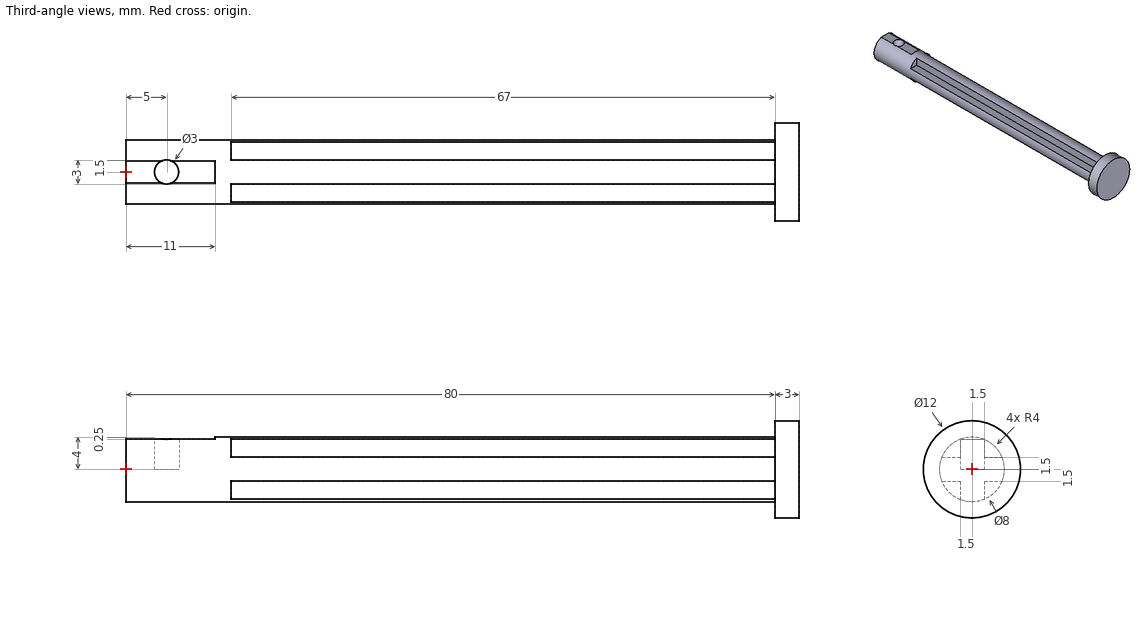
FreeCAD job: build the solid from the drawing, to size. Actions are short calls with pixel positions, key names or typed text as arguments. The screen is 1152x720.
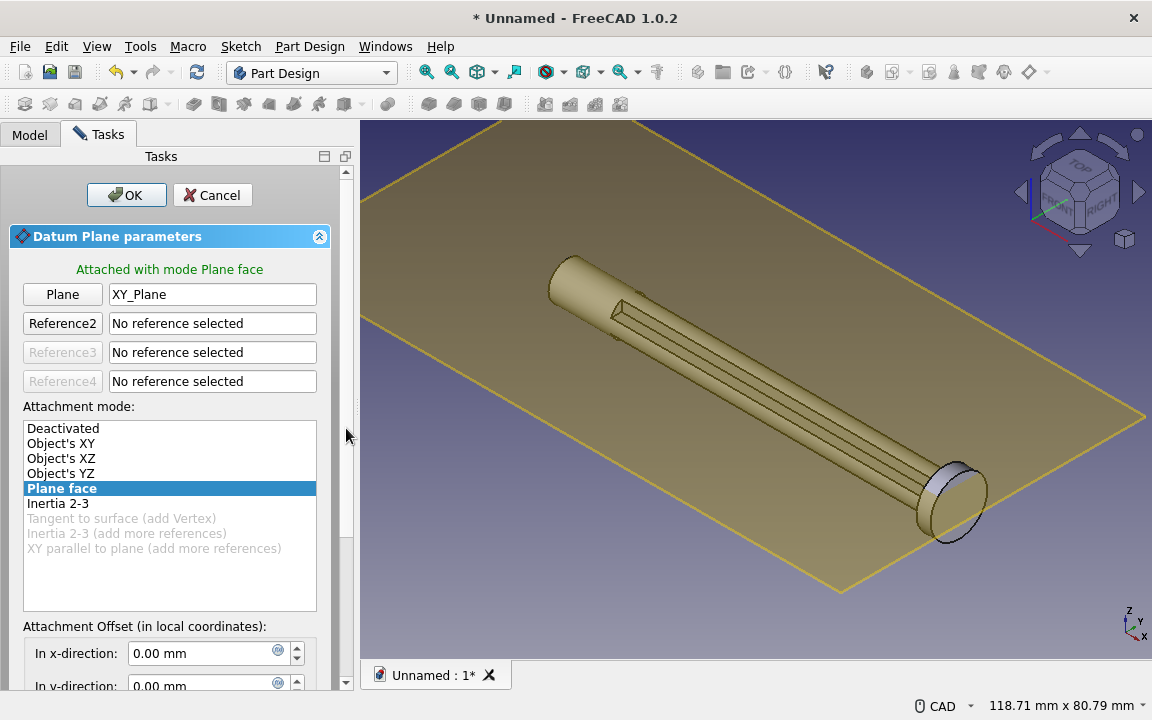
click(127, 195)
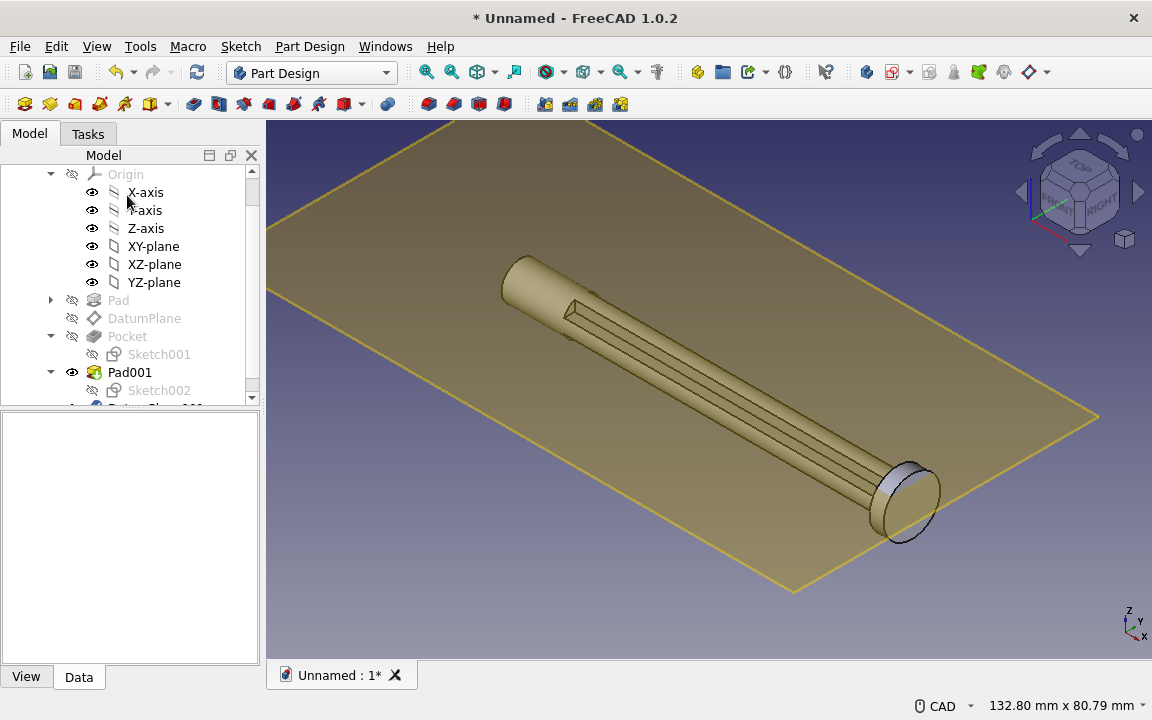
scroll(141, 278, down, 3)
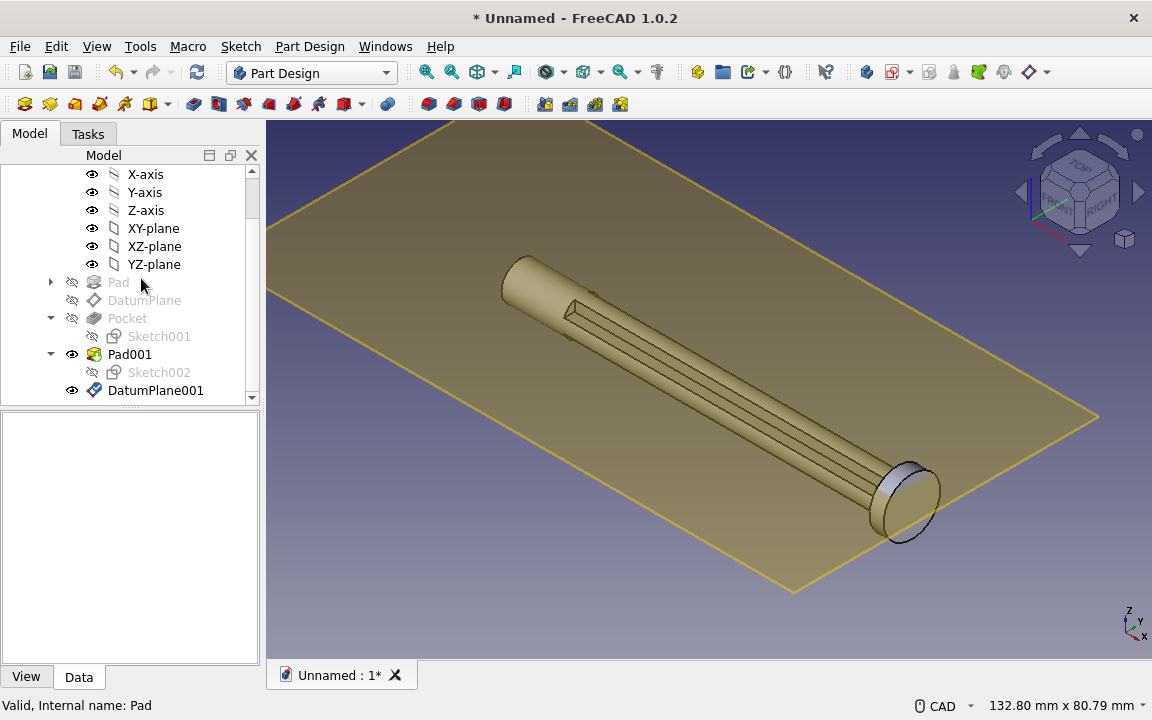
click(117, 390)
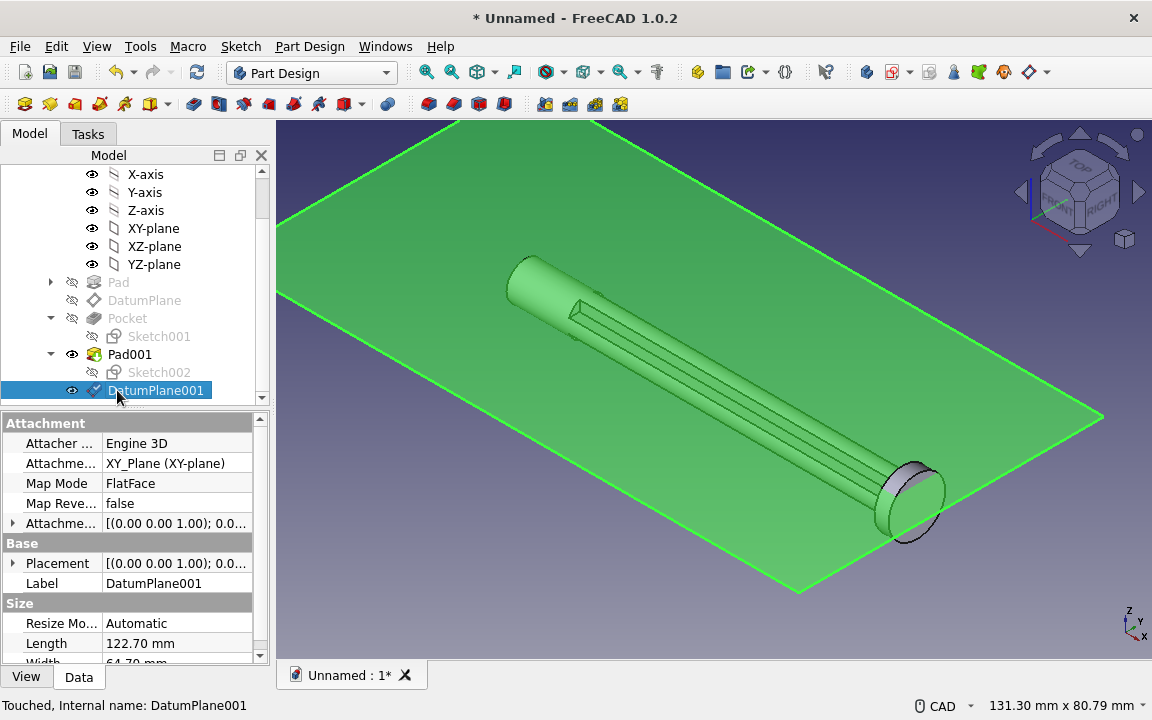
click(892, 72)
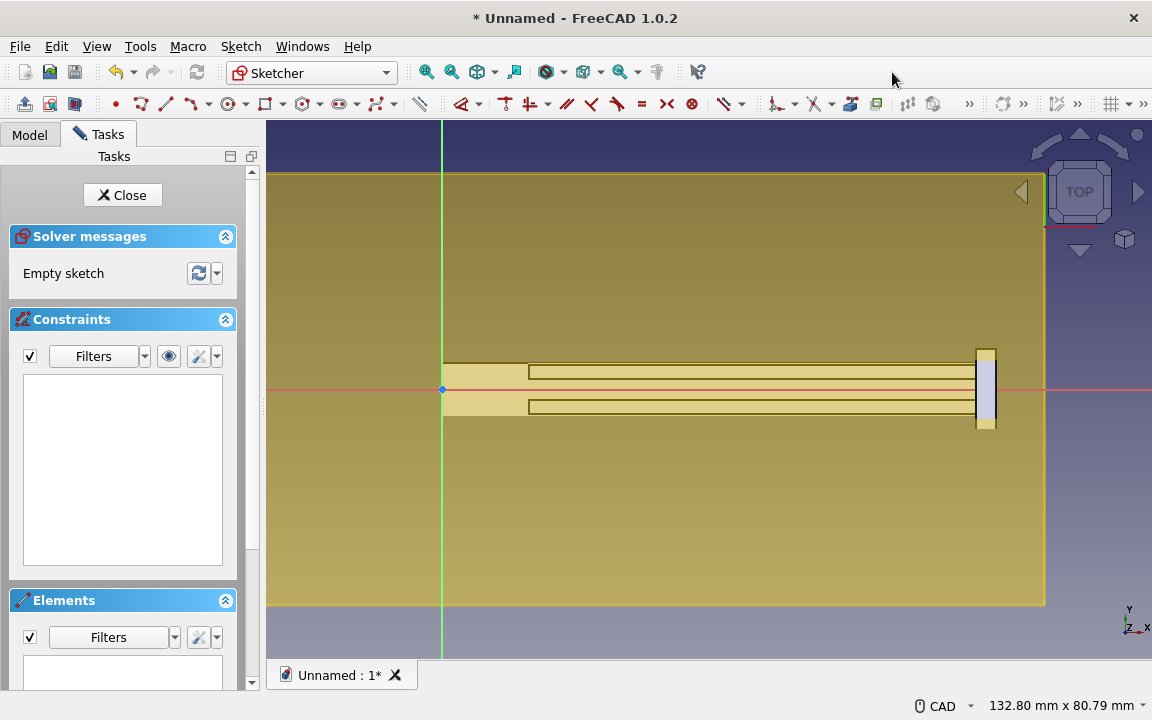
key(q)
key(s)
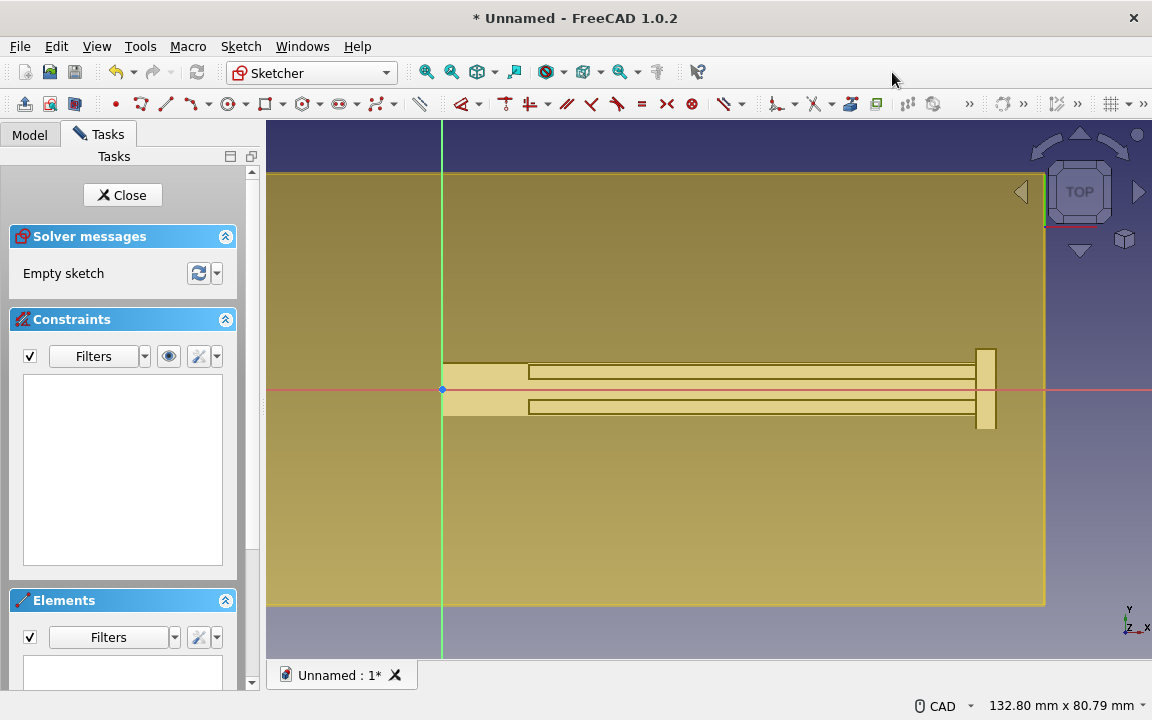
scroll(446, 390, up, 12)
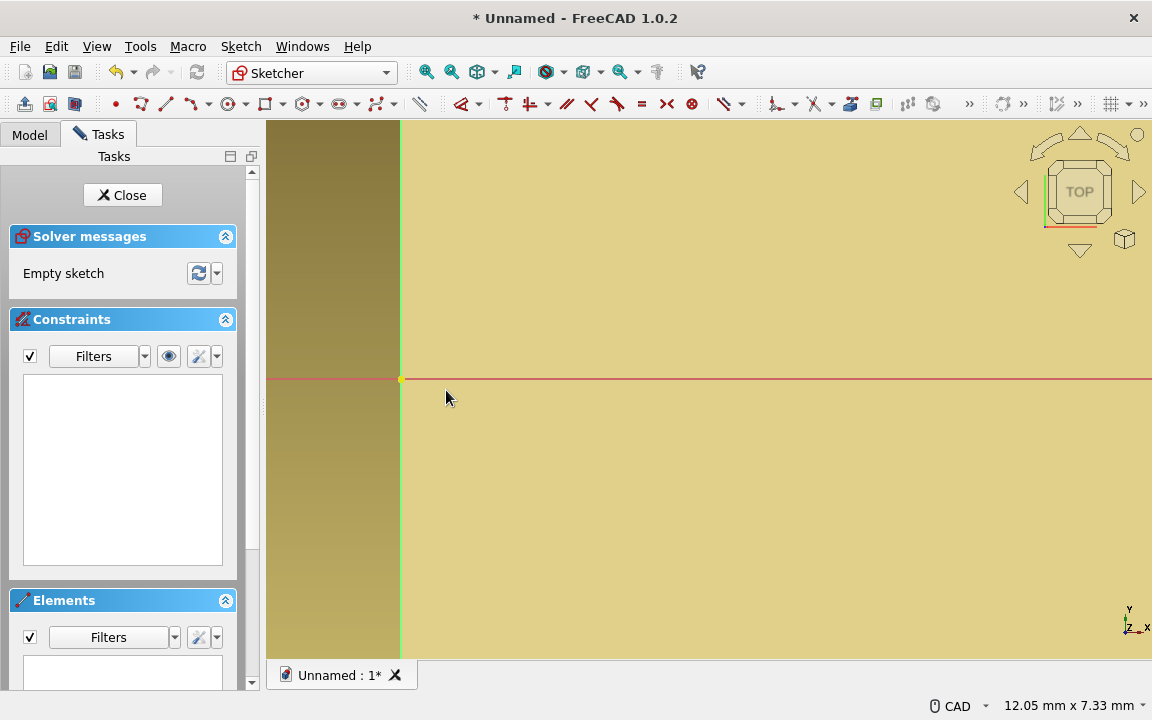
key(g)
key(c)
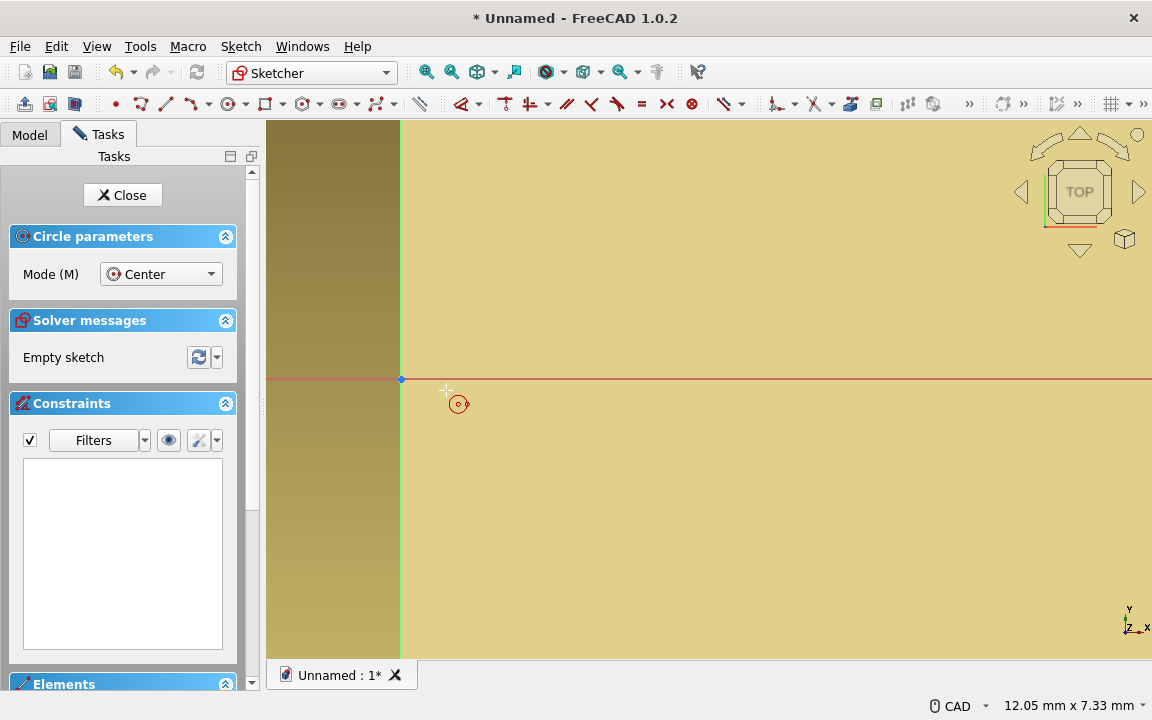
click(769, 379)
move(847, 301)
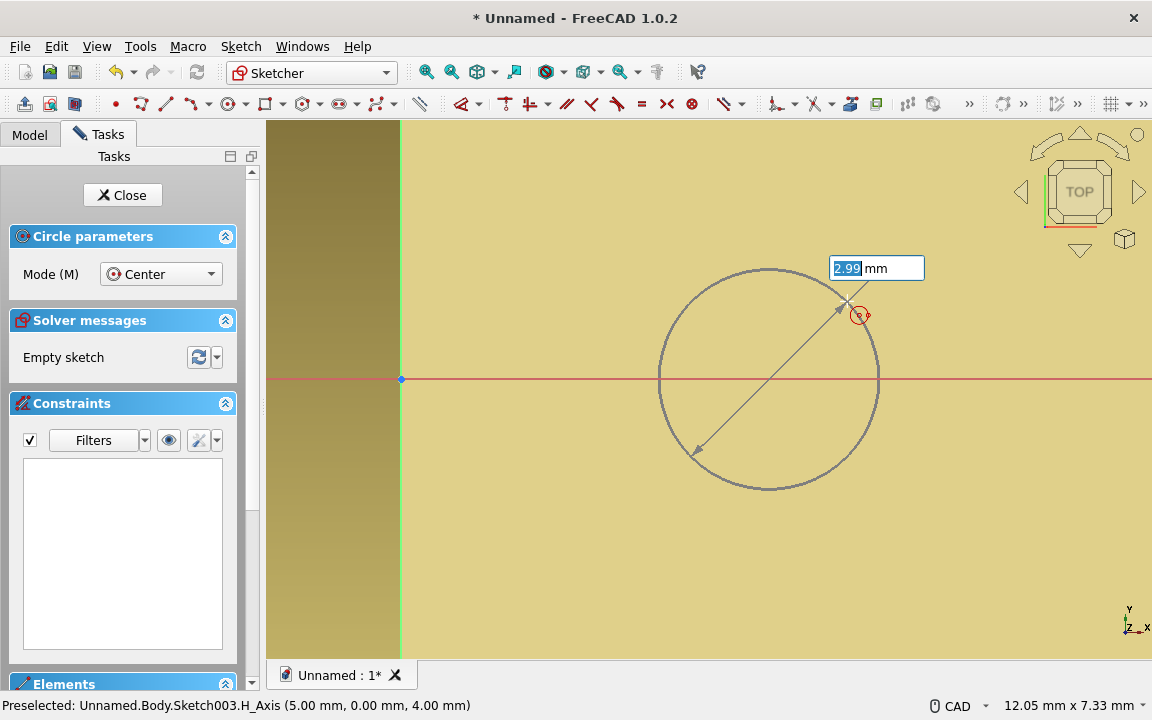
text(3)
key(Return)
key(Escape)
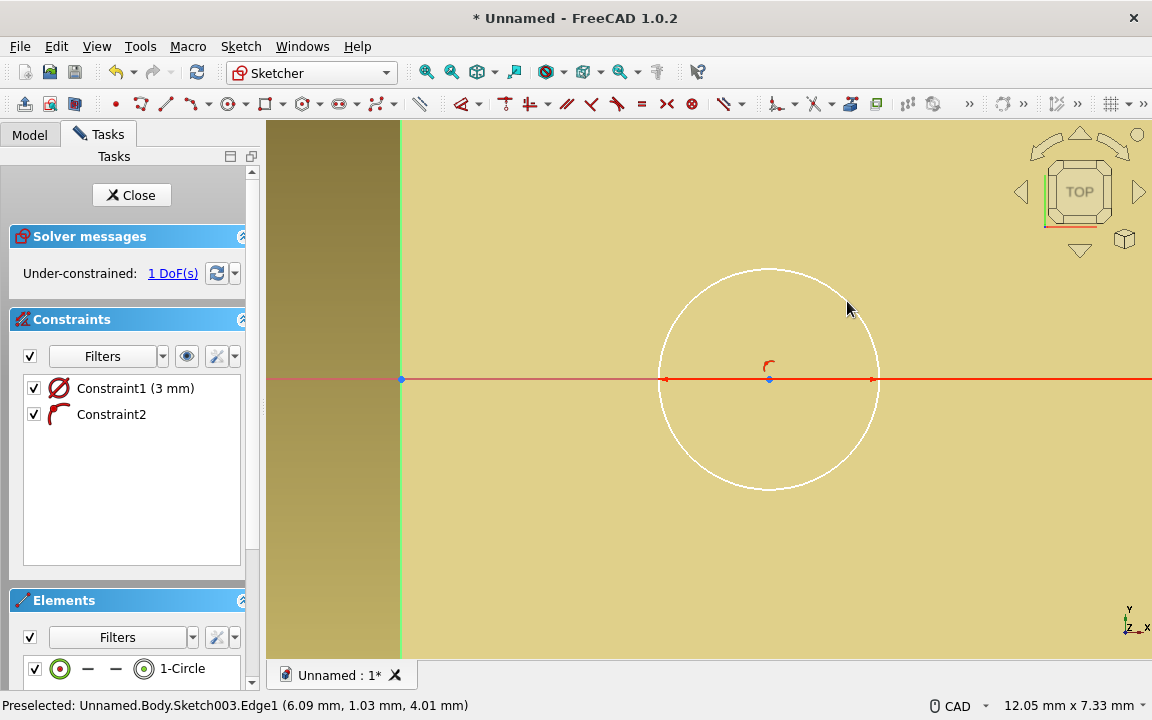
click(769, 379)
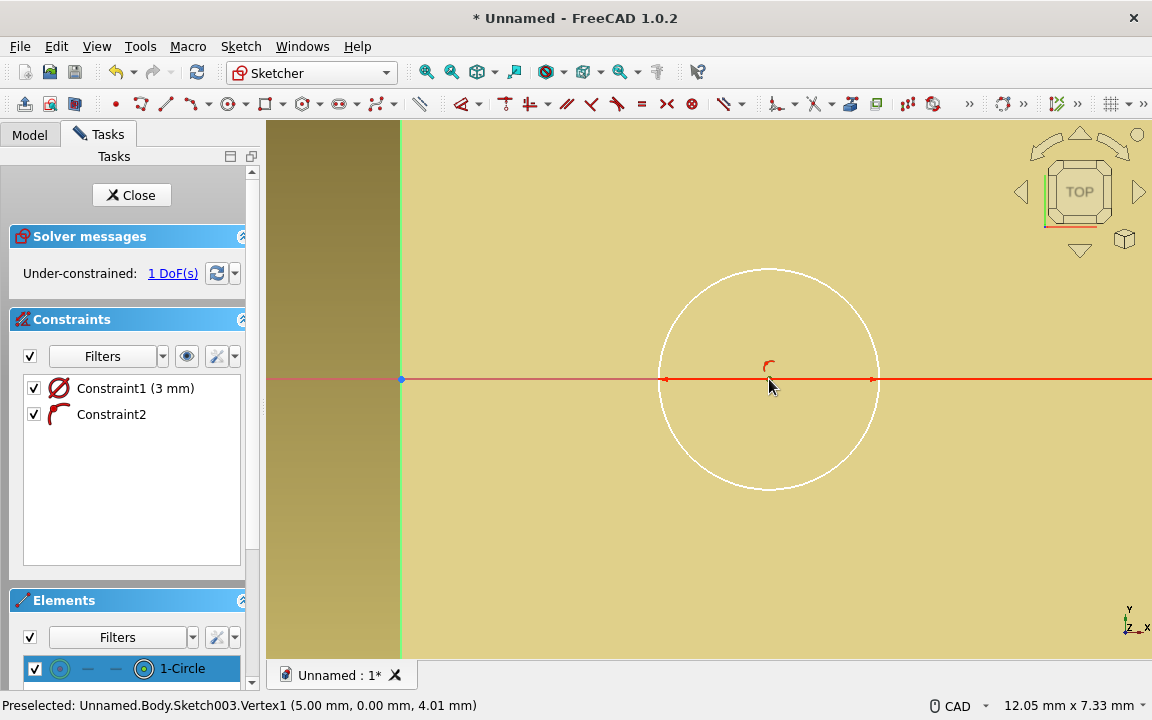
key(l)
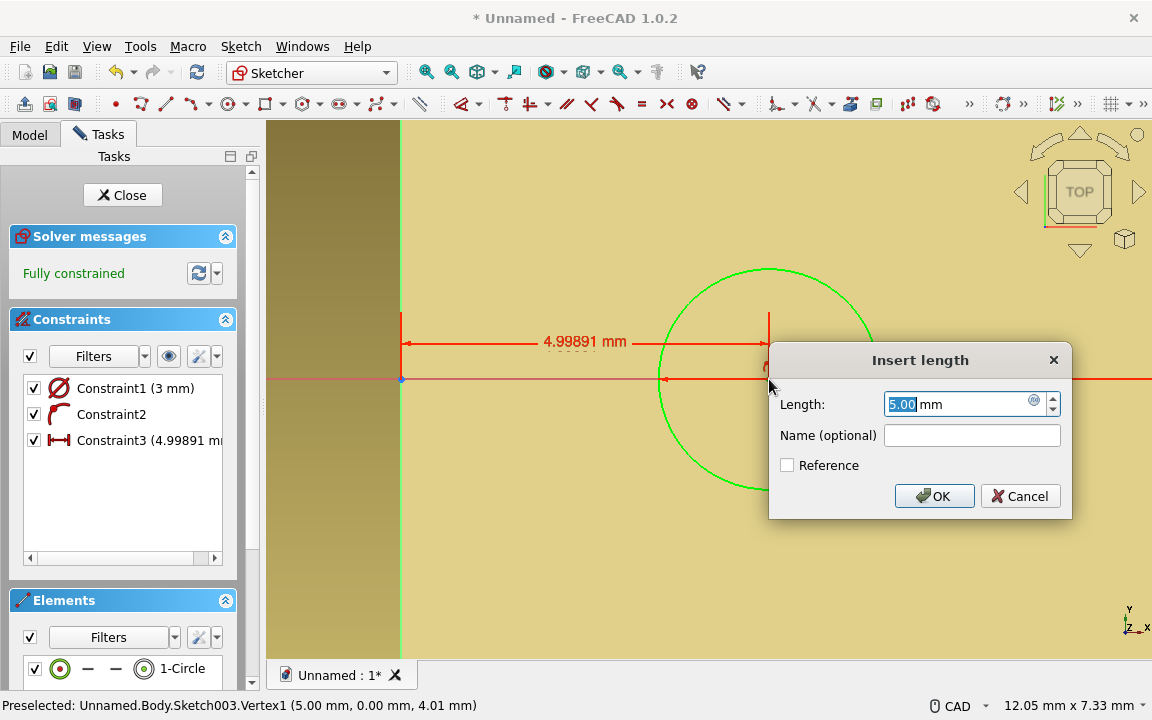
text(5)
key(Return)